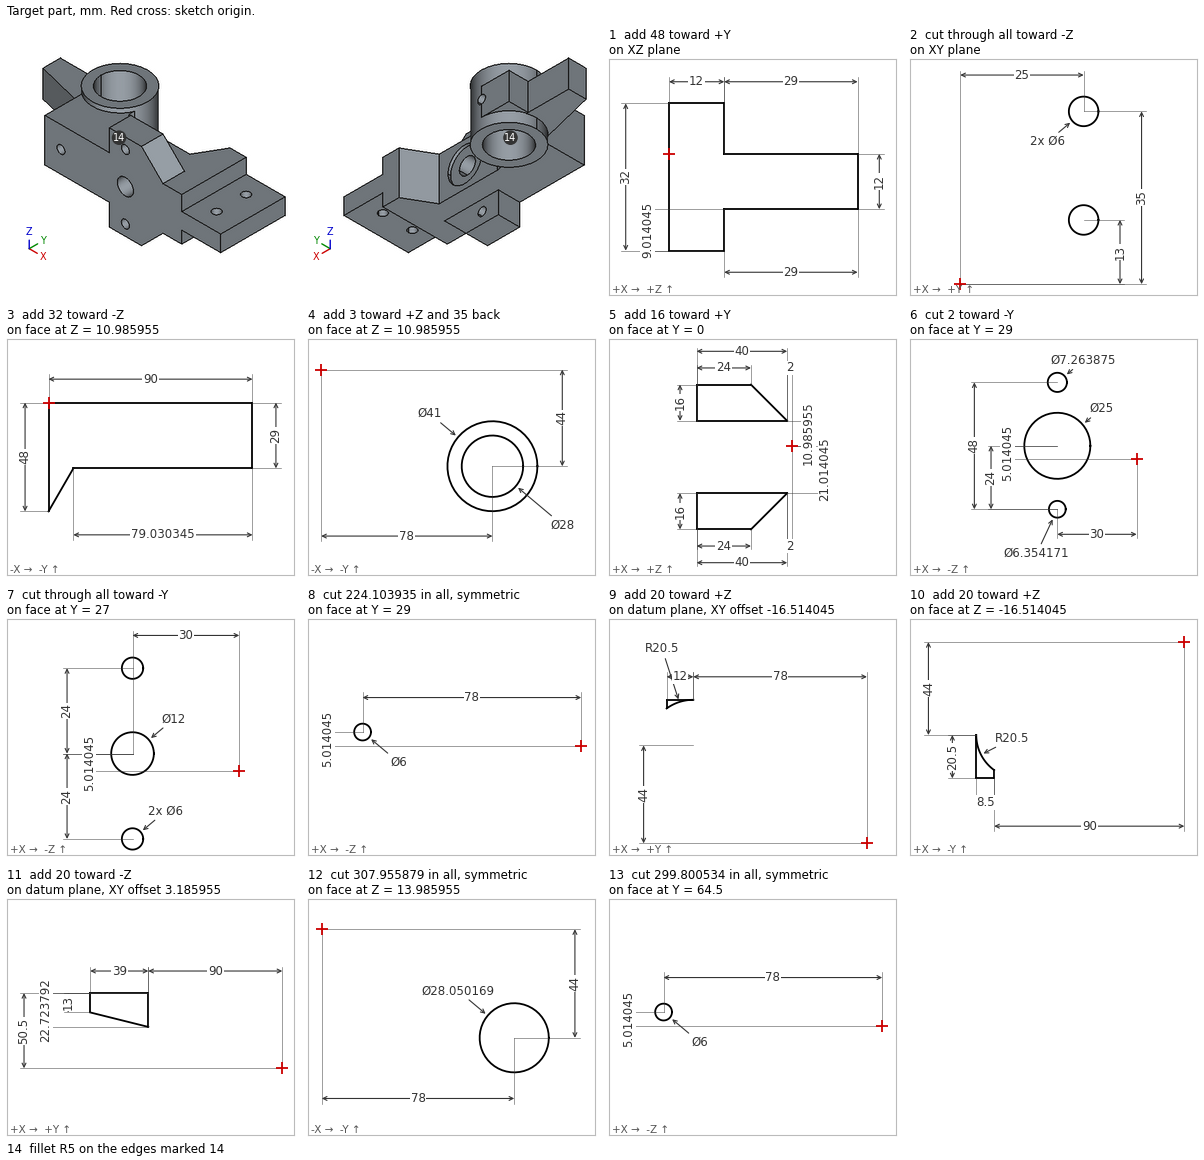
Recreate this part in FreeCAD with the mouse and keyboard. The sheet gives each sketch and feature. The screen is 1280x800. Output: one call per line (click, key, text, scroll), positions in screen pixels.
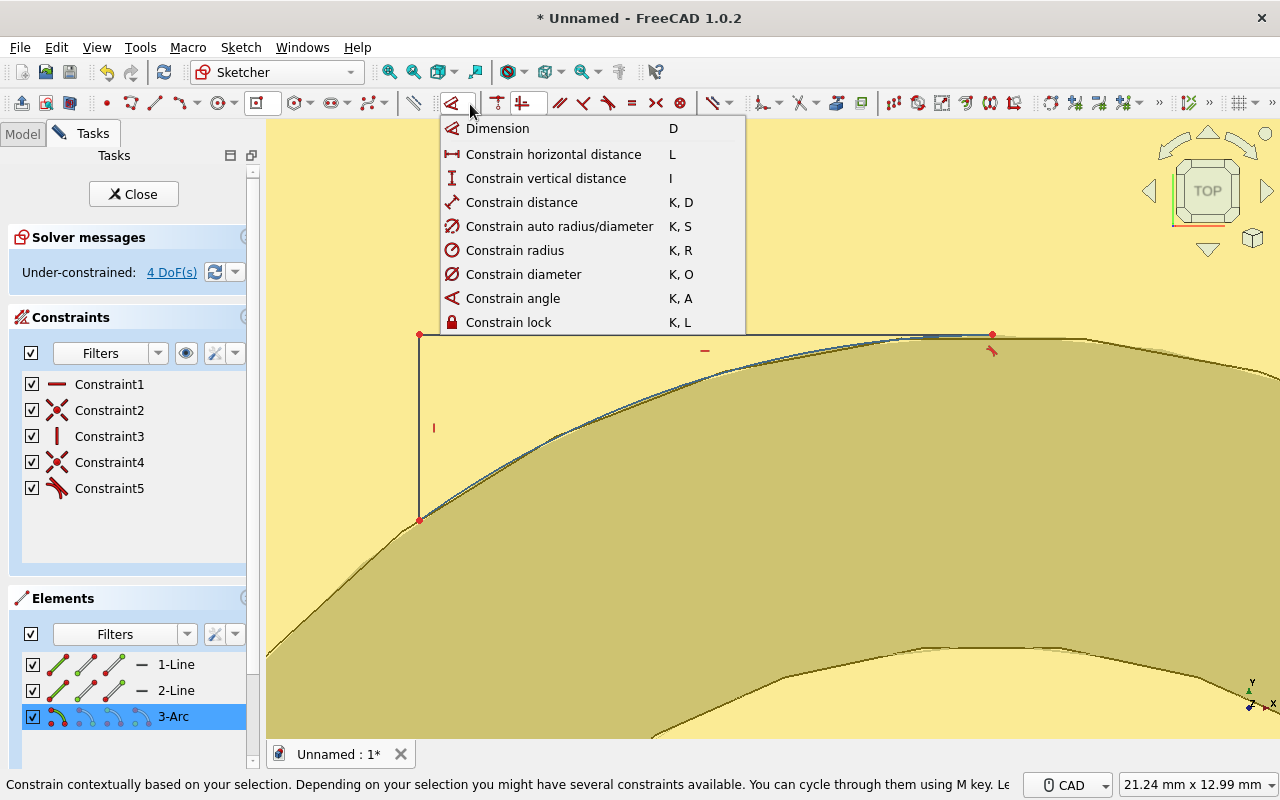
click(593, 250)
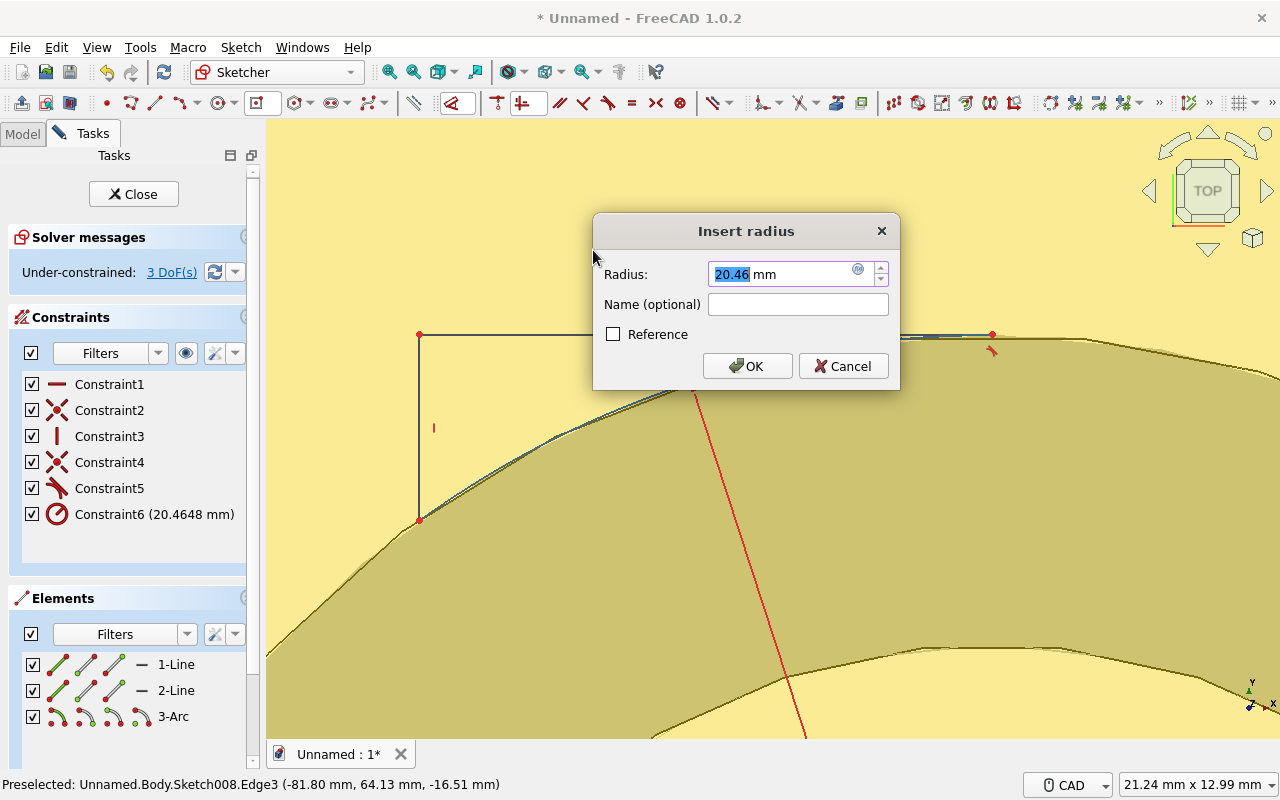
text(20.5)
key(Return)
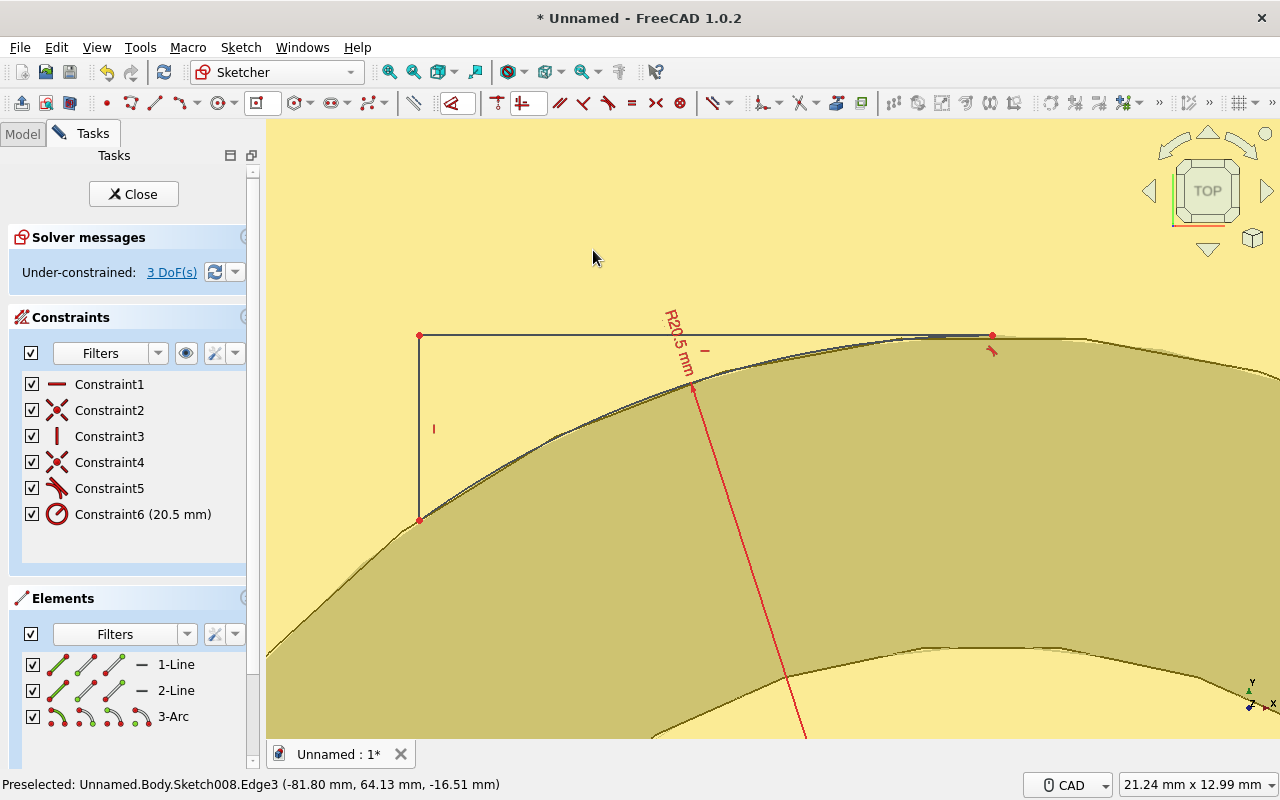
click(820, 335)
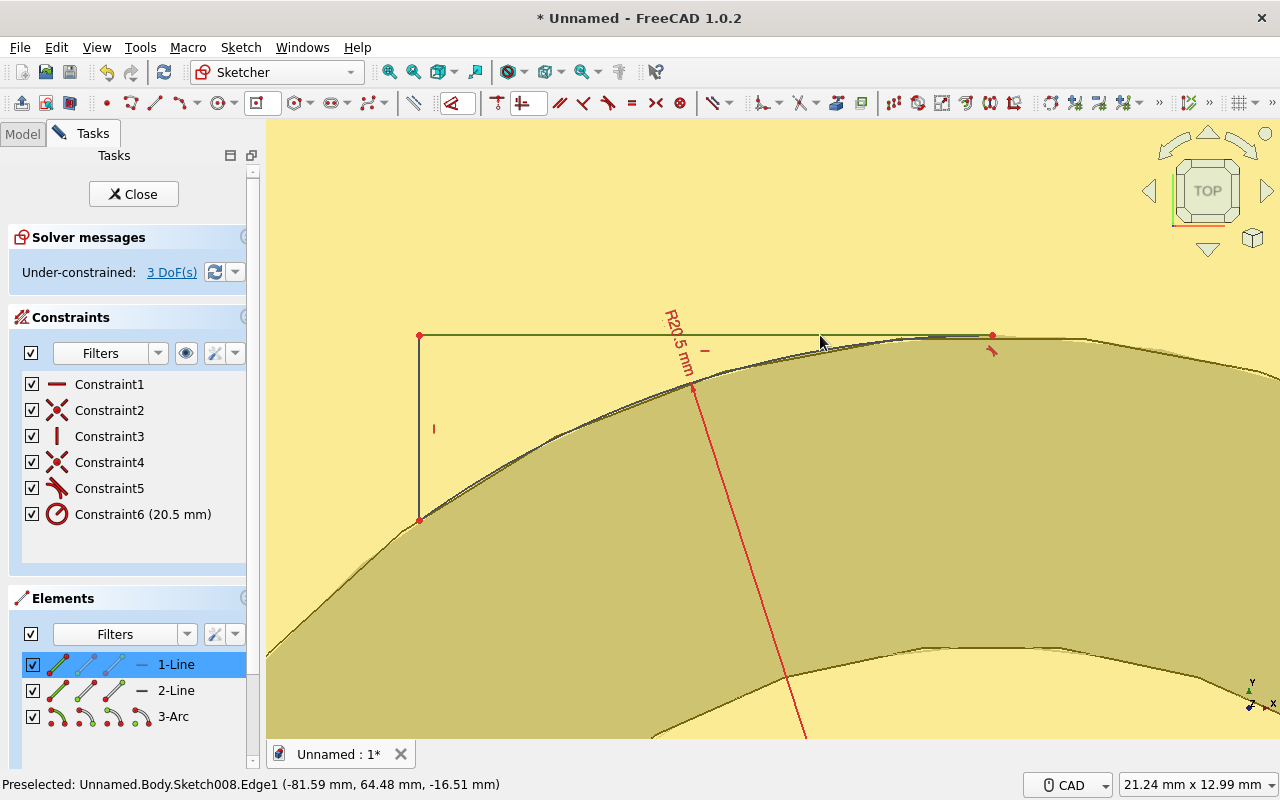
key(l)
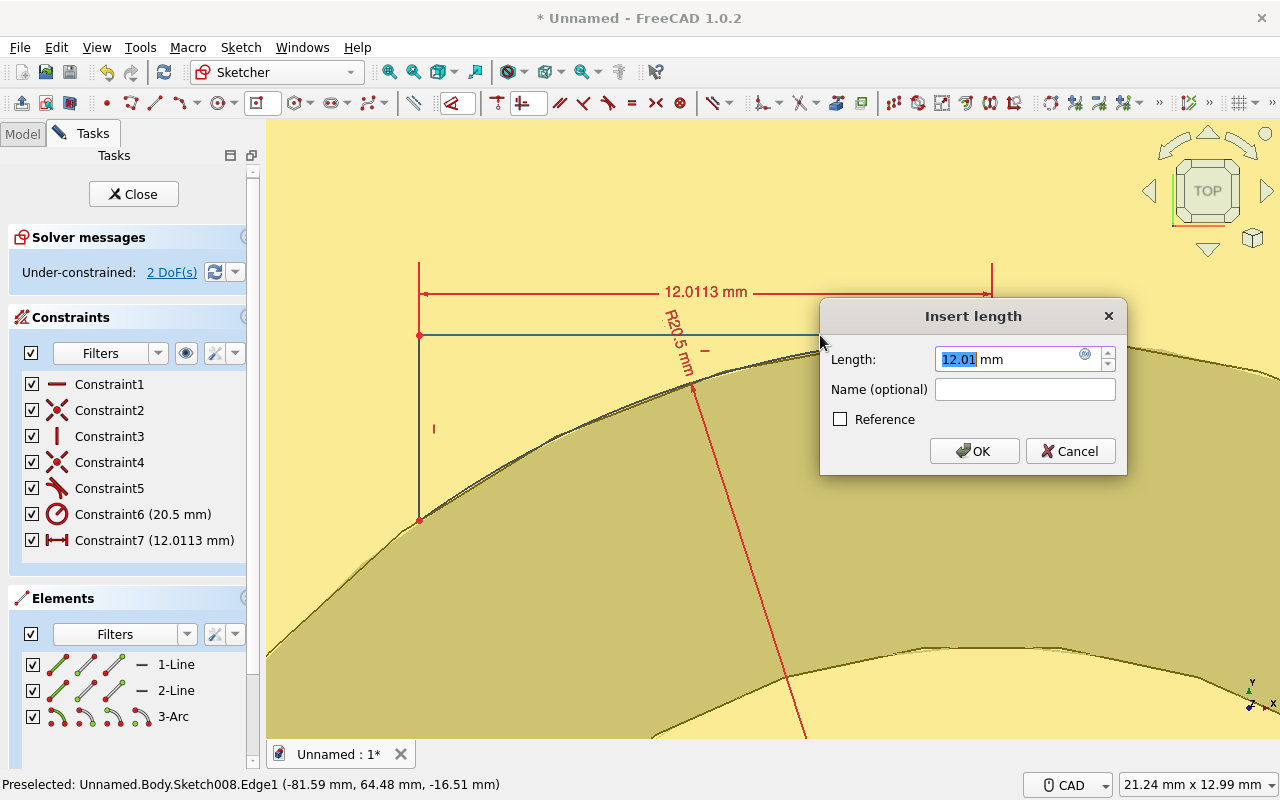
text(12)
key(Return)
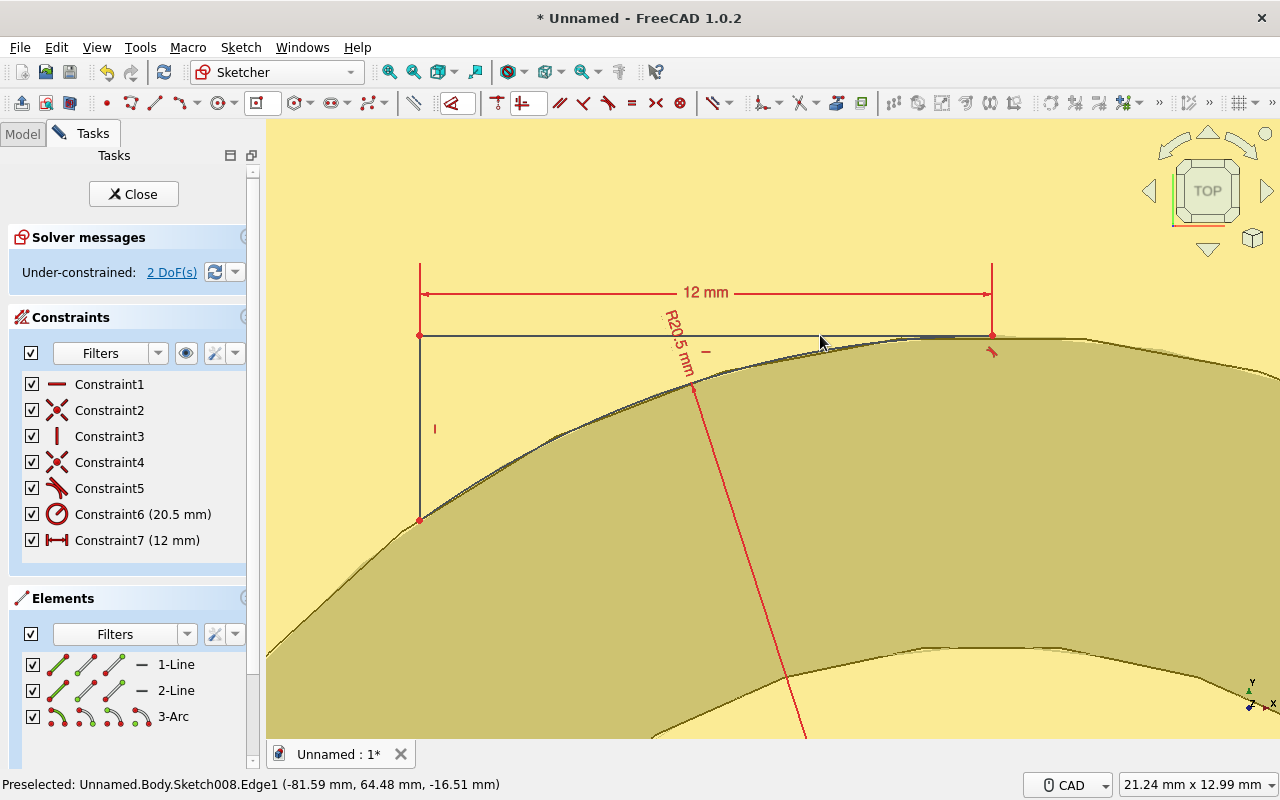
click(992, 336)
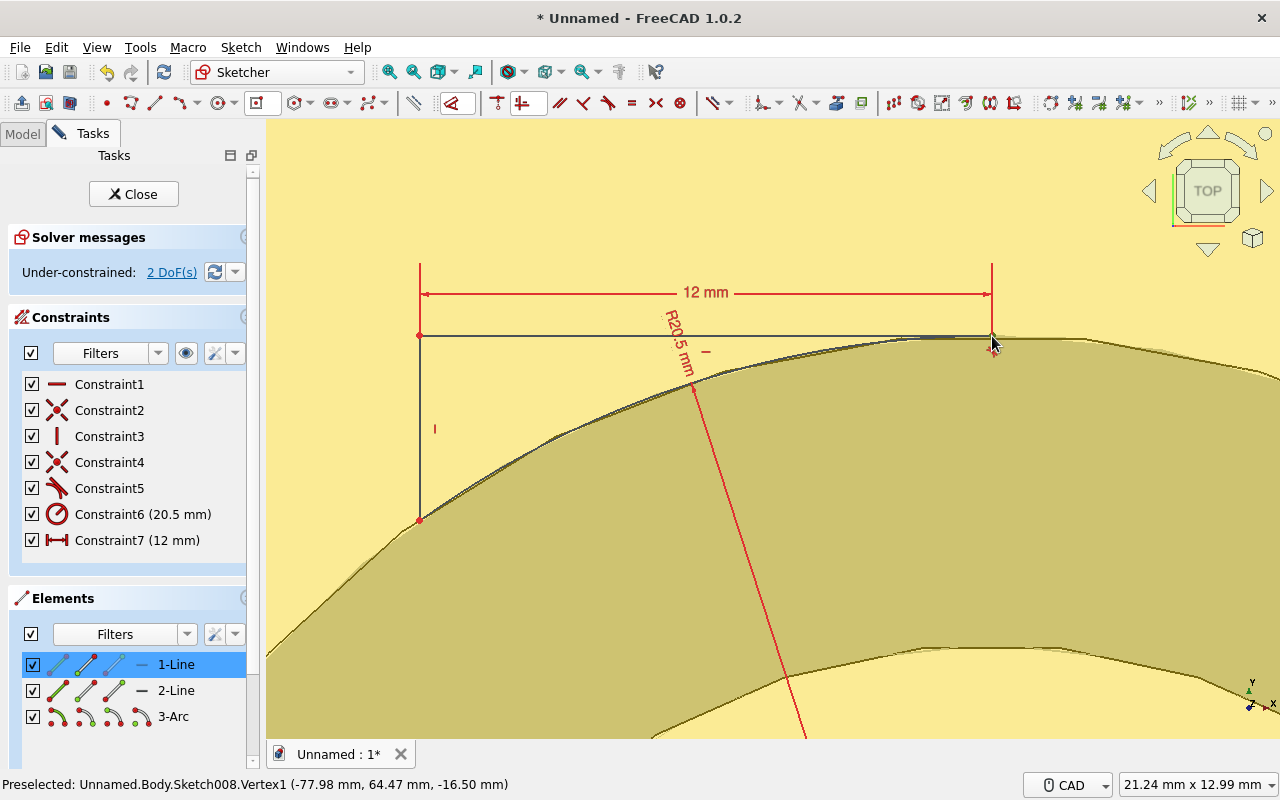
key(l)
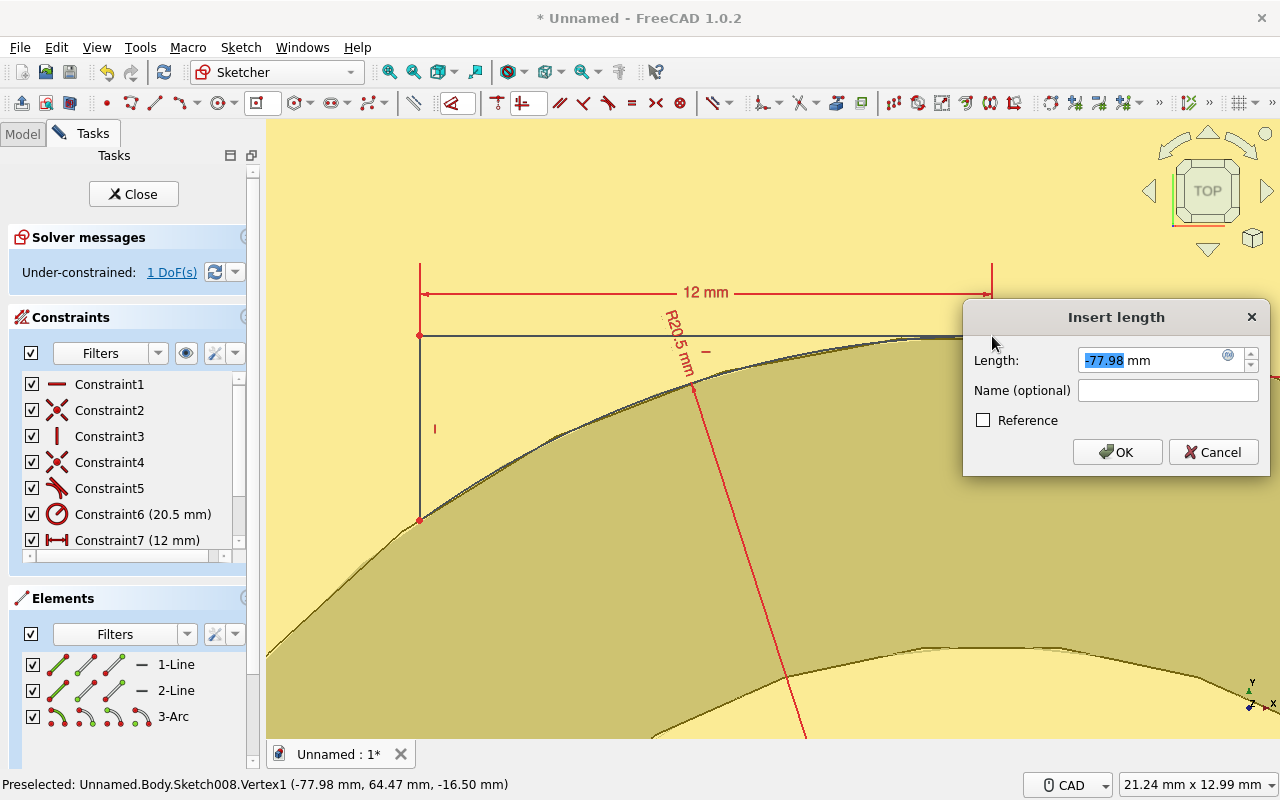
text(-78)
key(Return)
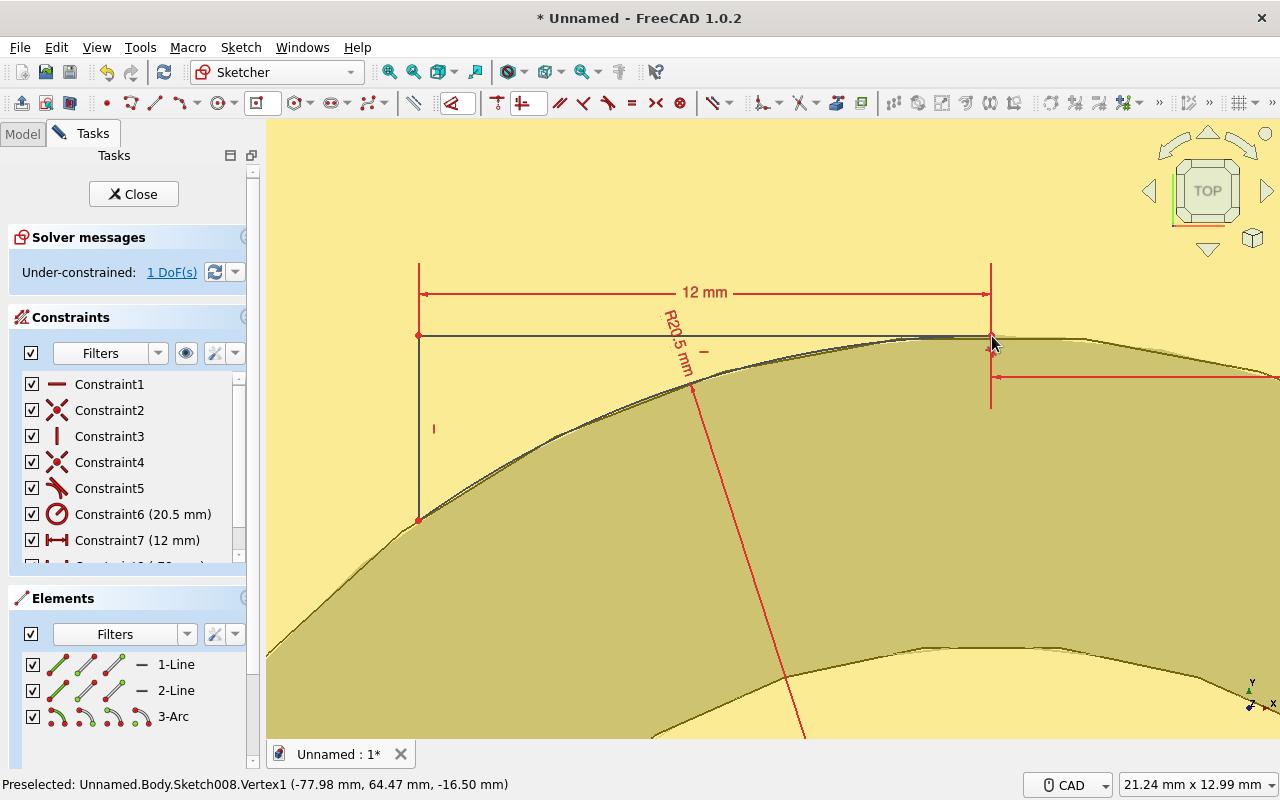
scroll(704, 199, down, 5)